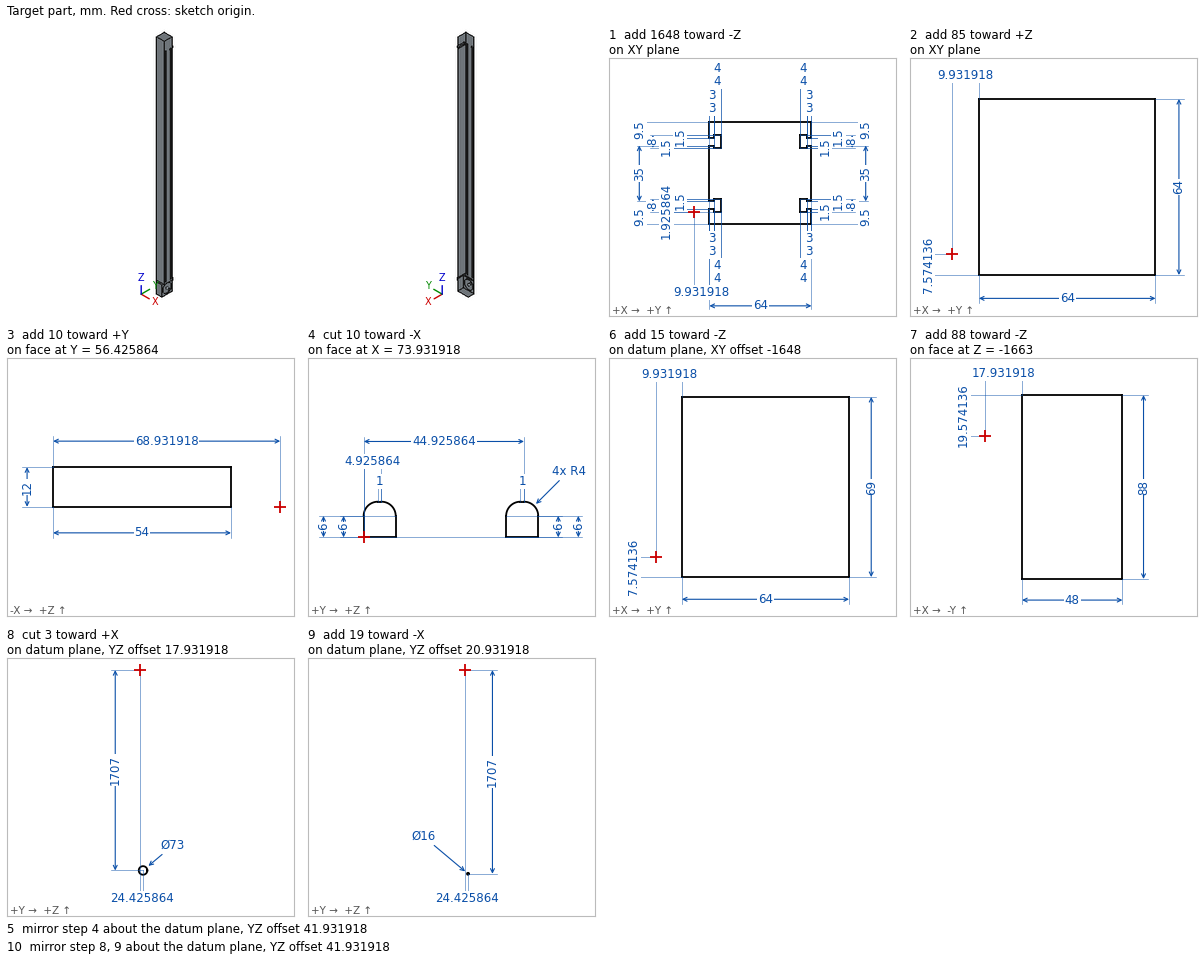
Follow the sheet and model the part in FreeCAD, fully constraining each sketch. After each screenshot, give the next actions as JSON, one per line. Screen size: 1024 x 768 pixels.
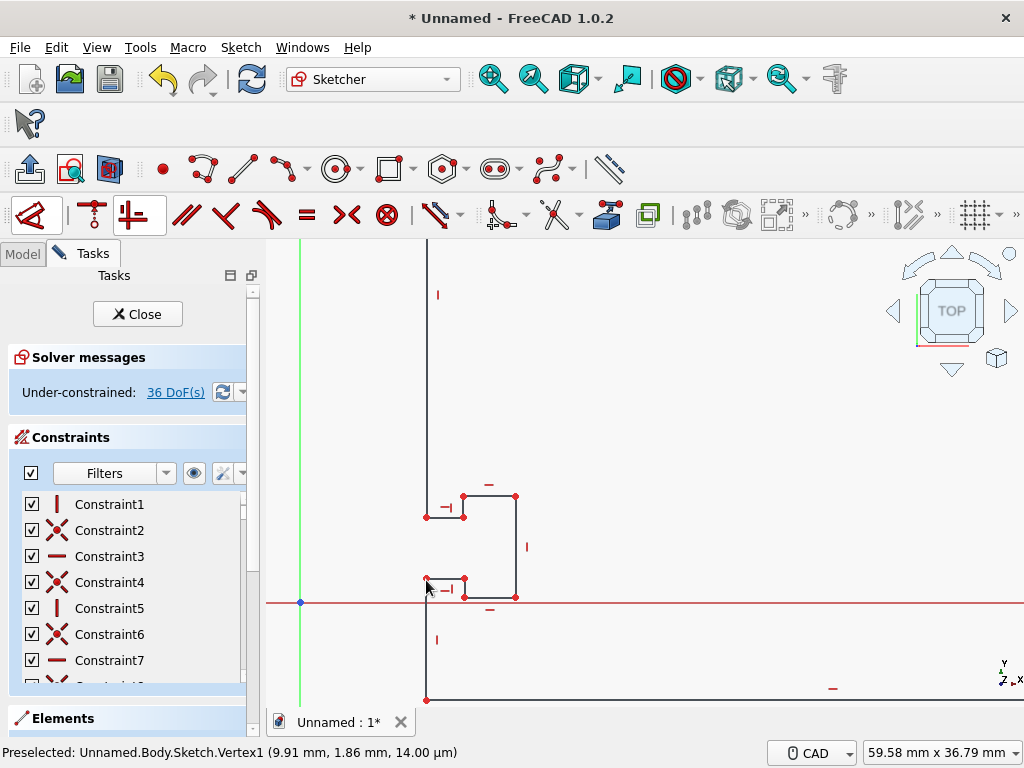
{"action": "left_click", "coordinate": [30, 216]}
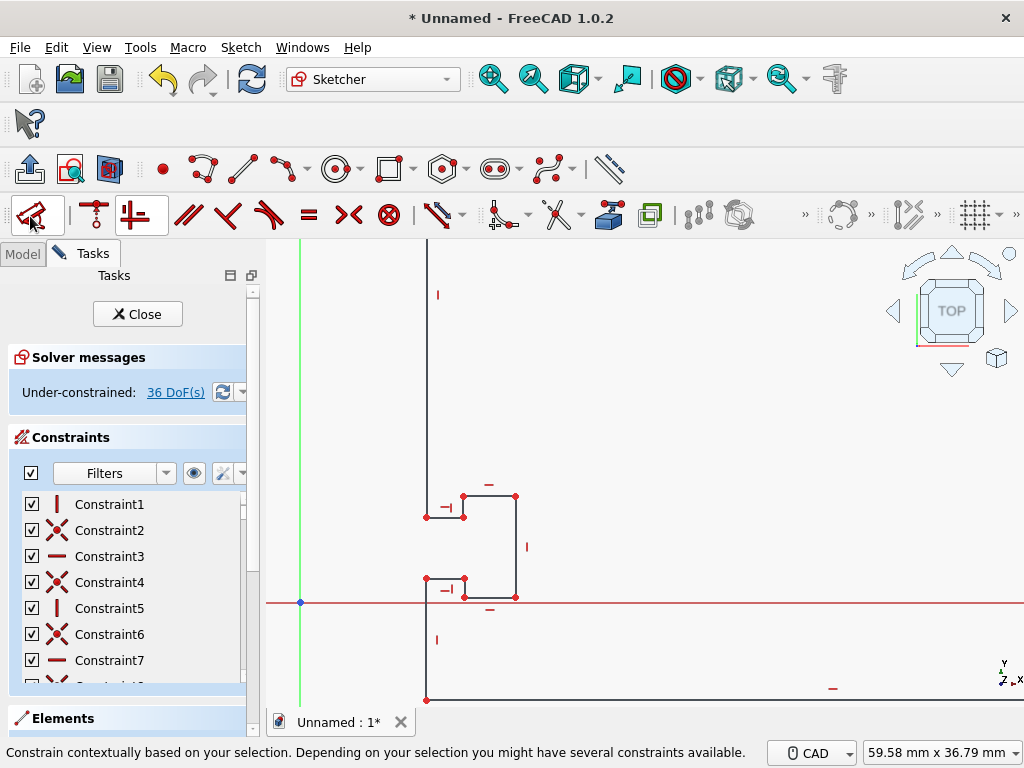
{"action": "scroll", "coordinate": [464, 578], "scroll_direction": "down", "scroll_amount": 5}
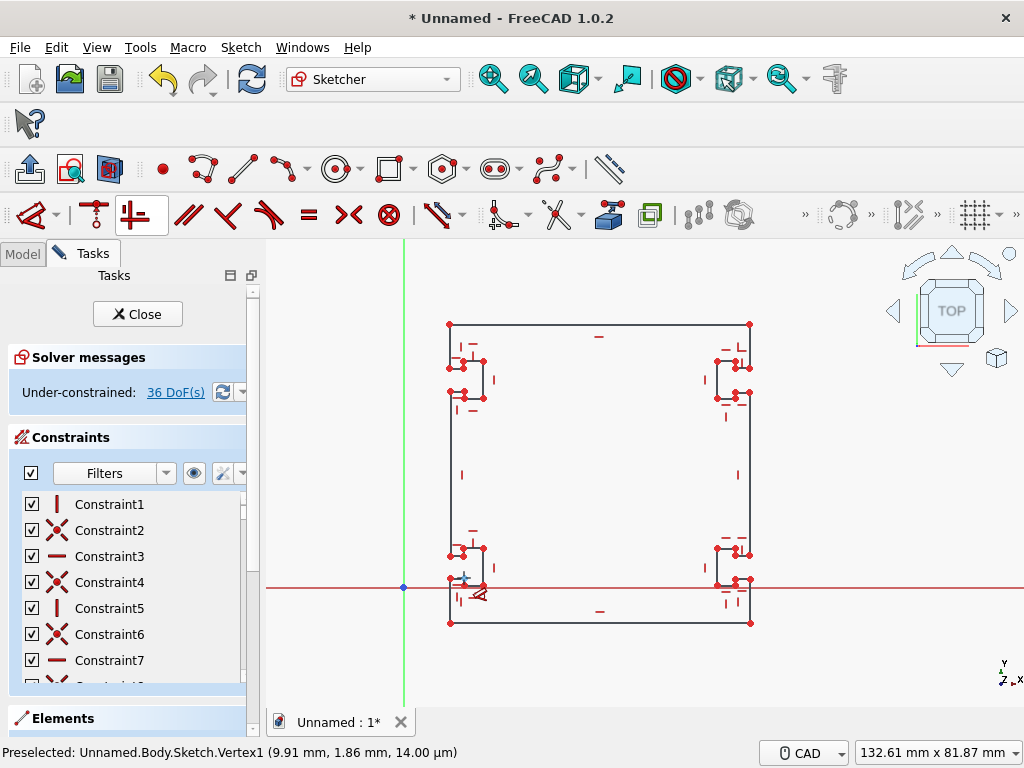
{"action": "scroll", "coordinate": [746, 579], "scroll_direction": "up", "scroll_amount": 6}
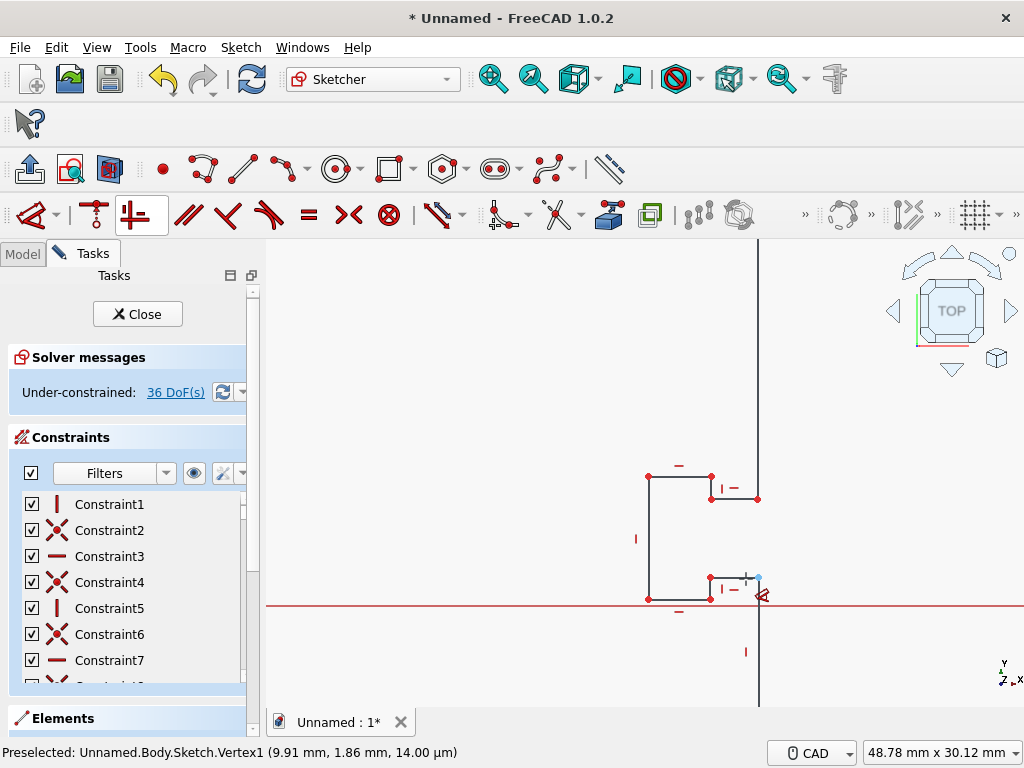
{"action": "left_click", "coordinate": [744, 578]}
{"action": "left_click", "coordinate": [734, 544]}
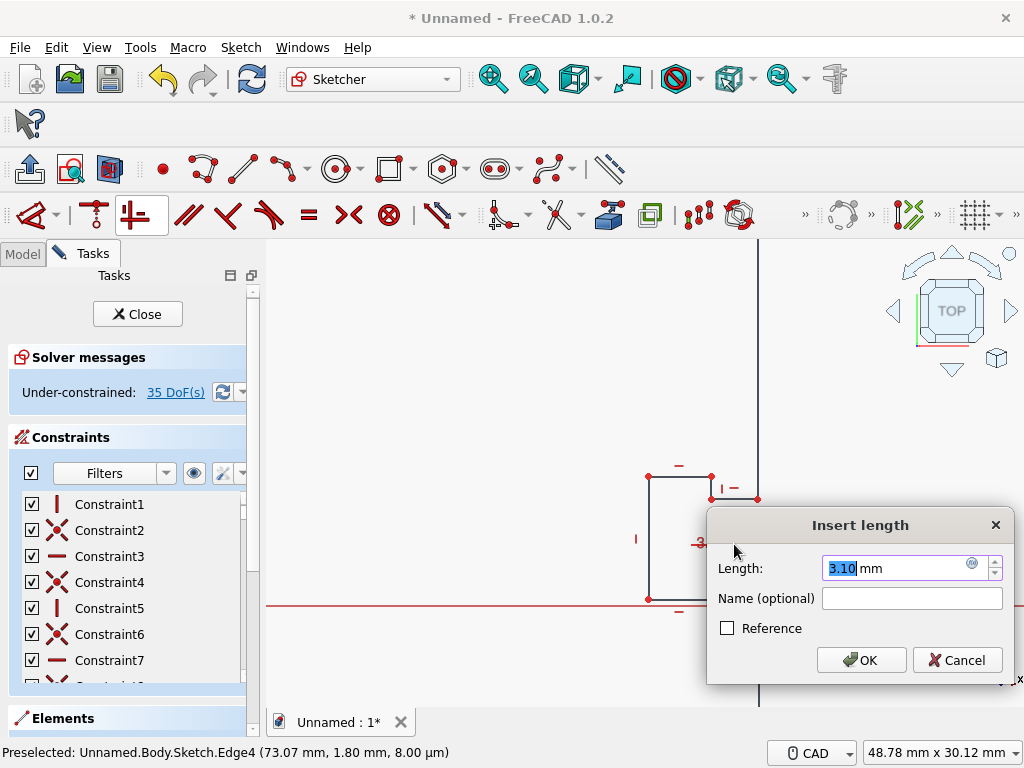
{"action": "type", "text": "3"}
{"action": "key", "text": "Return"}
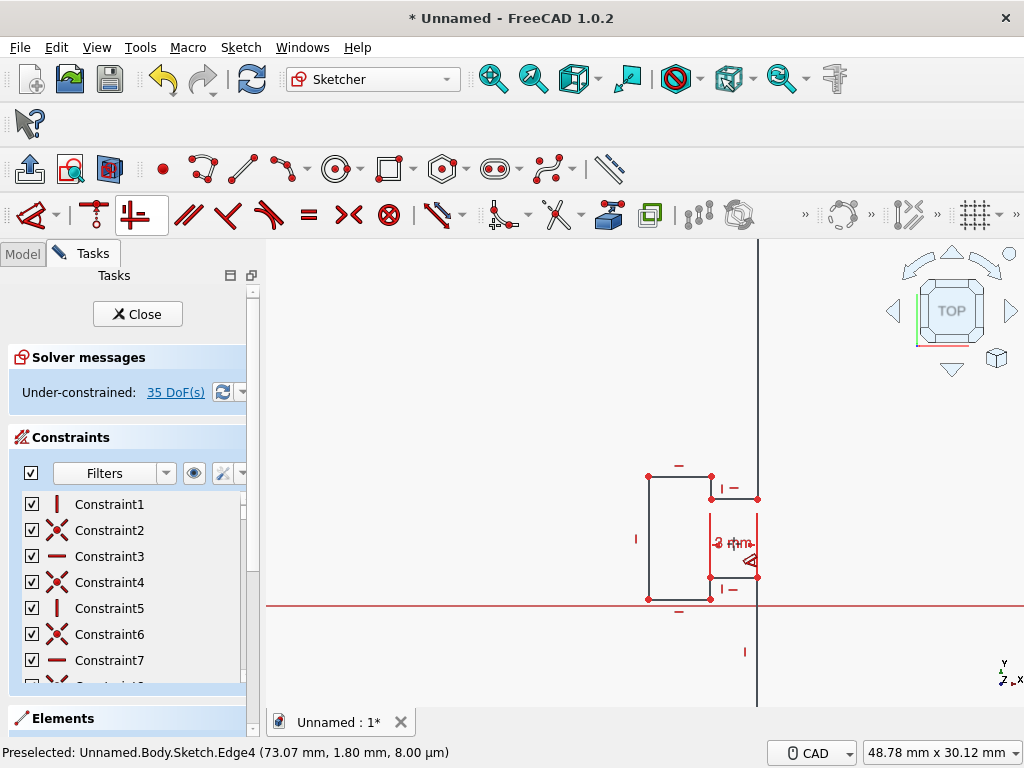
{"action": "scroll", "coordinate": [692, 600], "scroll_direction": "up", "scroll_amount": 5}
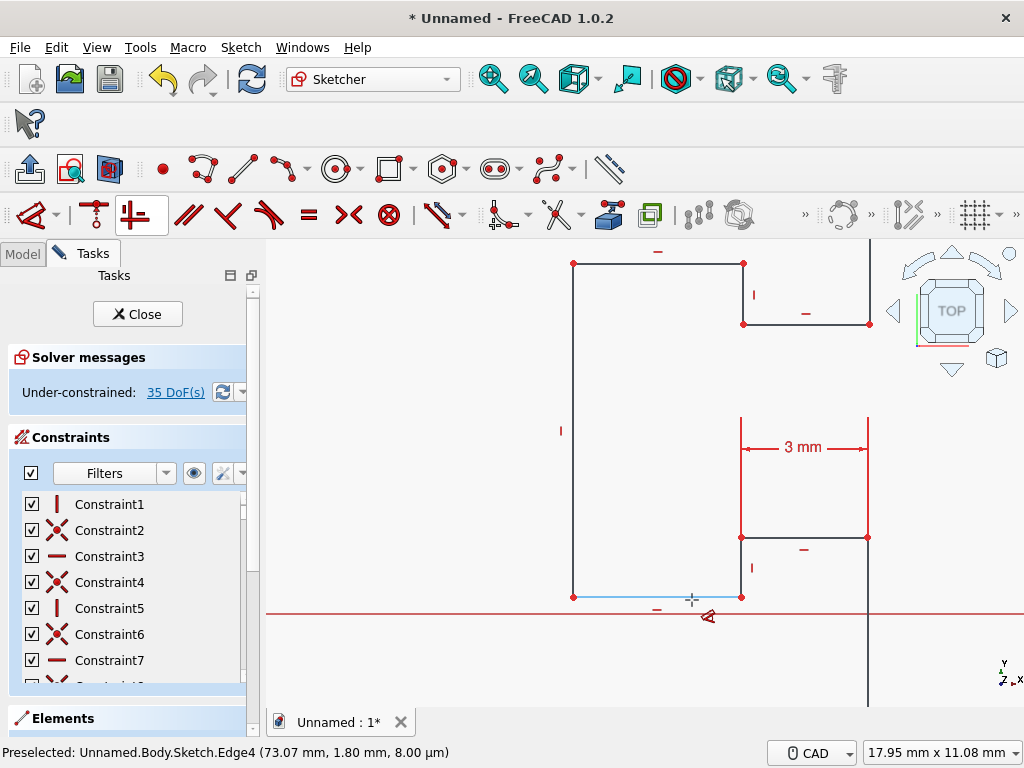
{"action": "left_click", "coordinate": [691, 597]}
{"action": "left_click", "coordinate": [657, 631]}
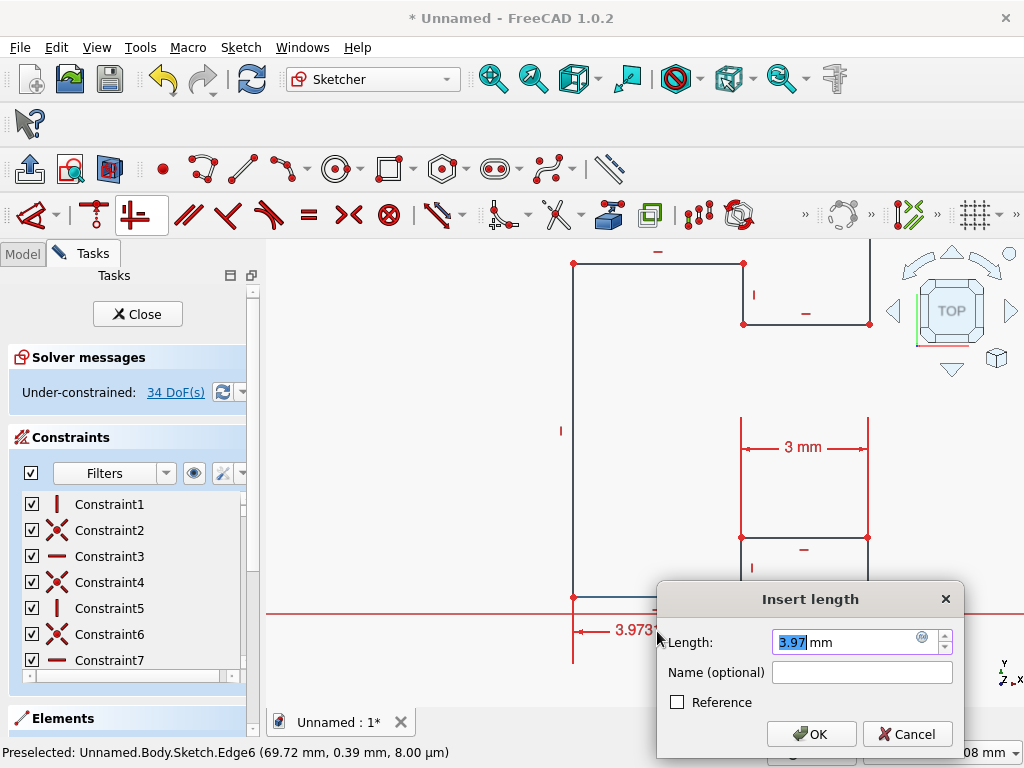
{"action": "type", "text": "4"}
{"action": "key", "text": "Return"}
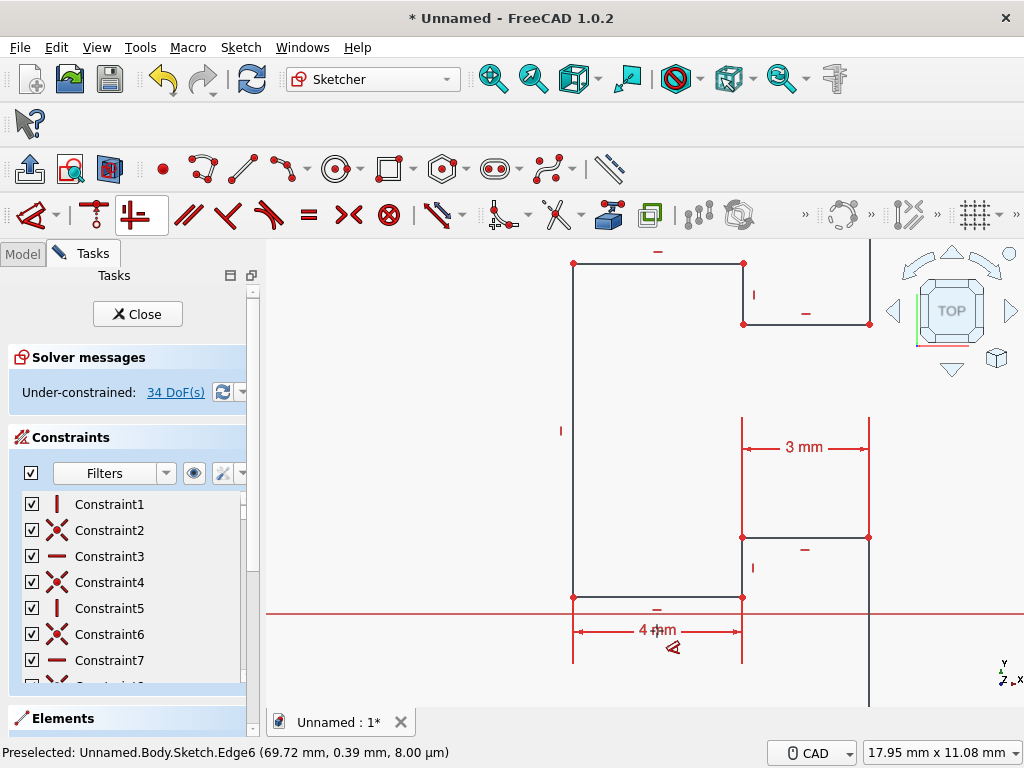
{"action": "scroll", "coordinate": [735, 584], "scroll_direction": "down", "scroll_amount": 11}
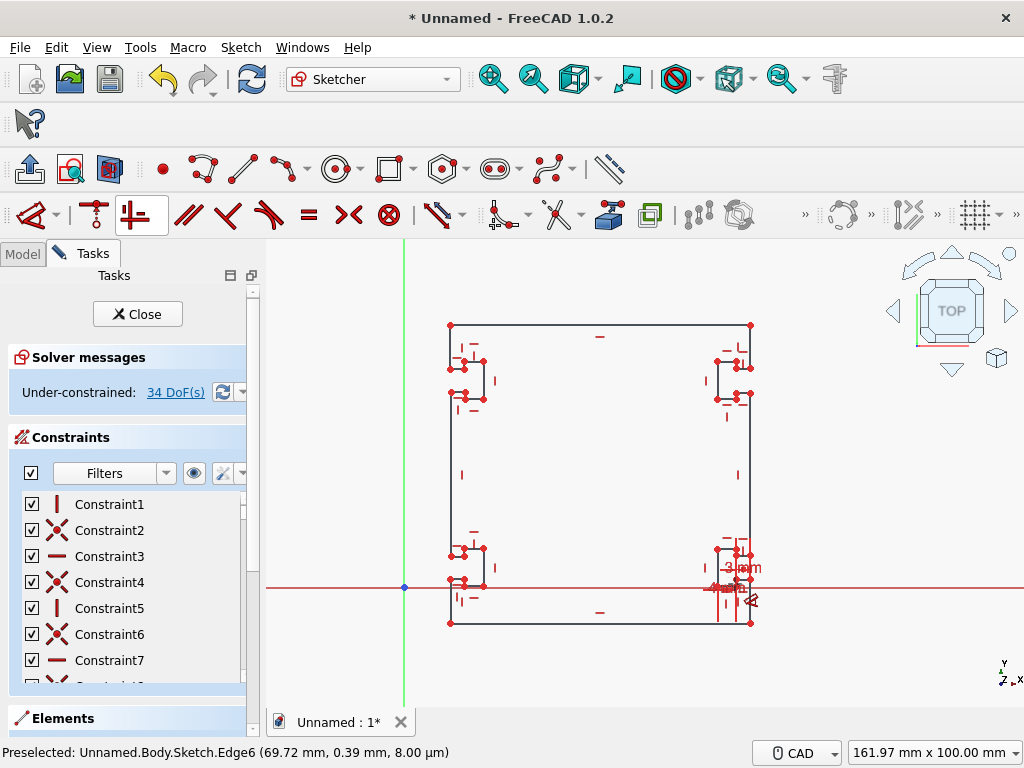
{"action": "scroll", "coordinate": [718, 575], "scroll_direction": "up", "scroll_amount": 2}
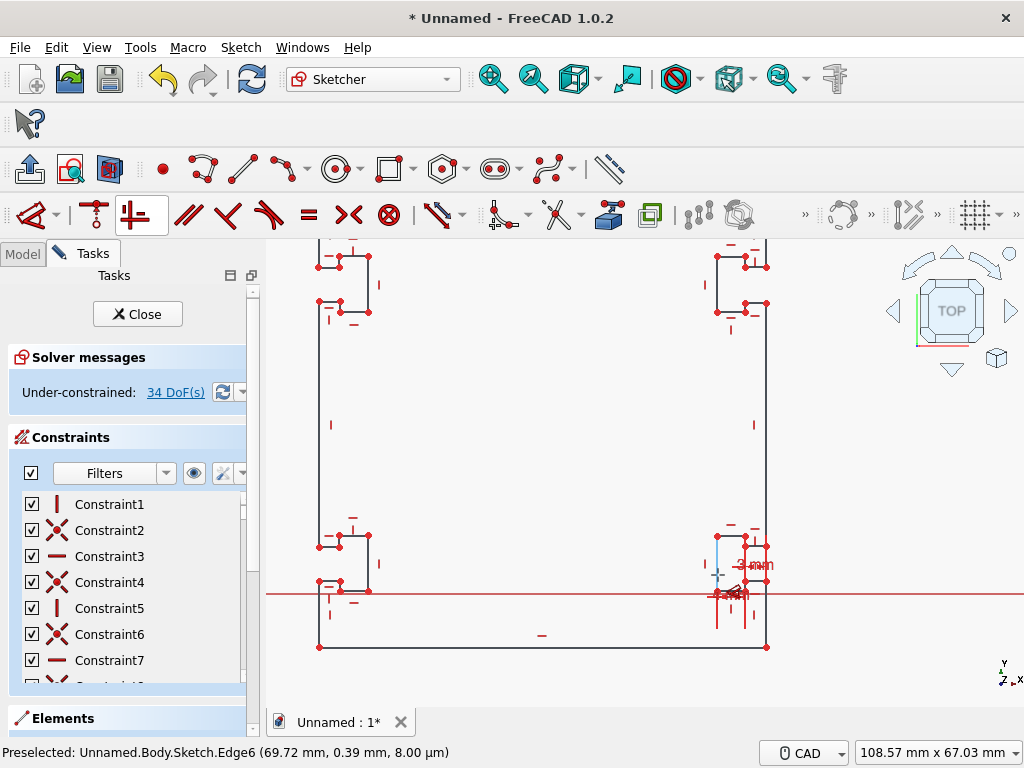
{"action": "left_click", "coordinate": [717, 575]}
{"action": "left_click", "coordinate": [683, 564]}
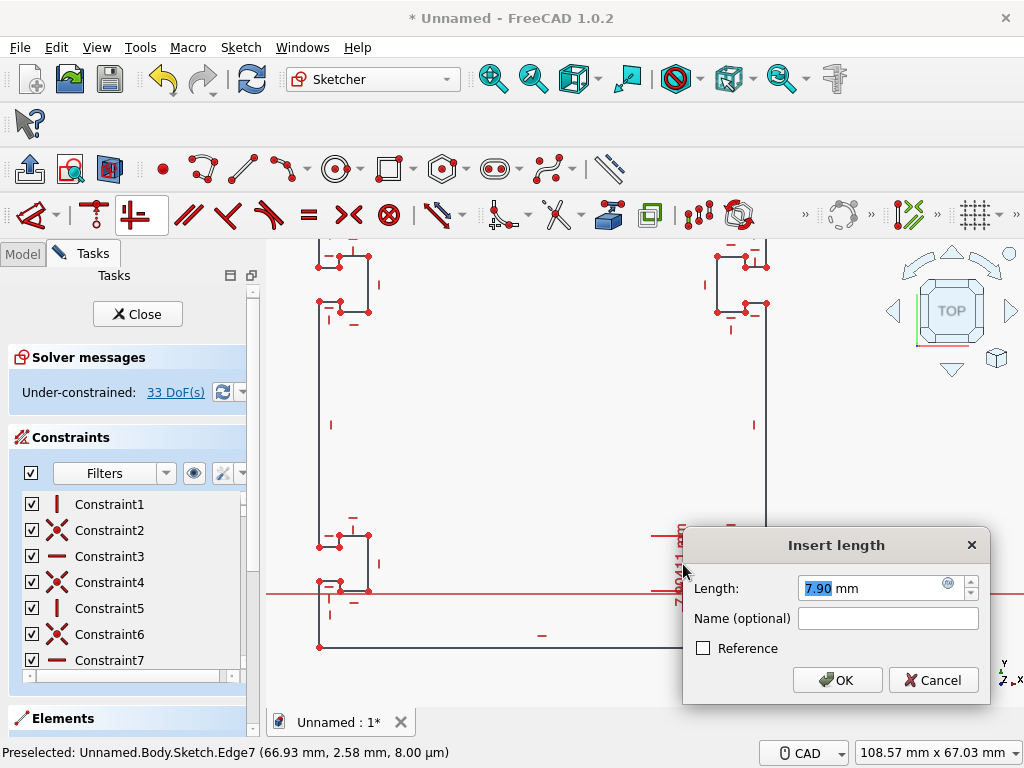
{"action": "type", "text": "8"}
{"action": "key", "text": "Return"}